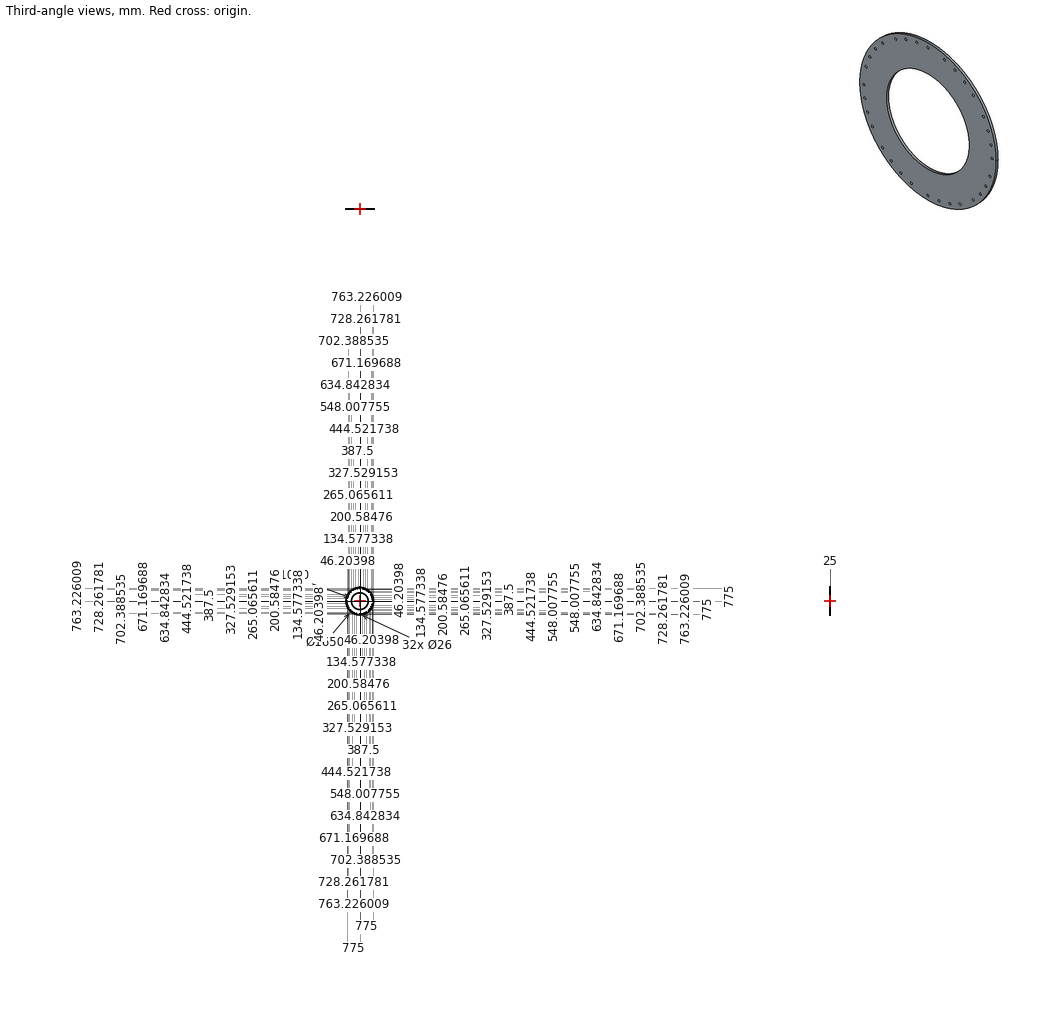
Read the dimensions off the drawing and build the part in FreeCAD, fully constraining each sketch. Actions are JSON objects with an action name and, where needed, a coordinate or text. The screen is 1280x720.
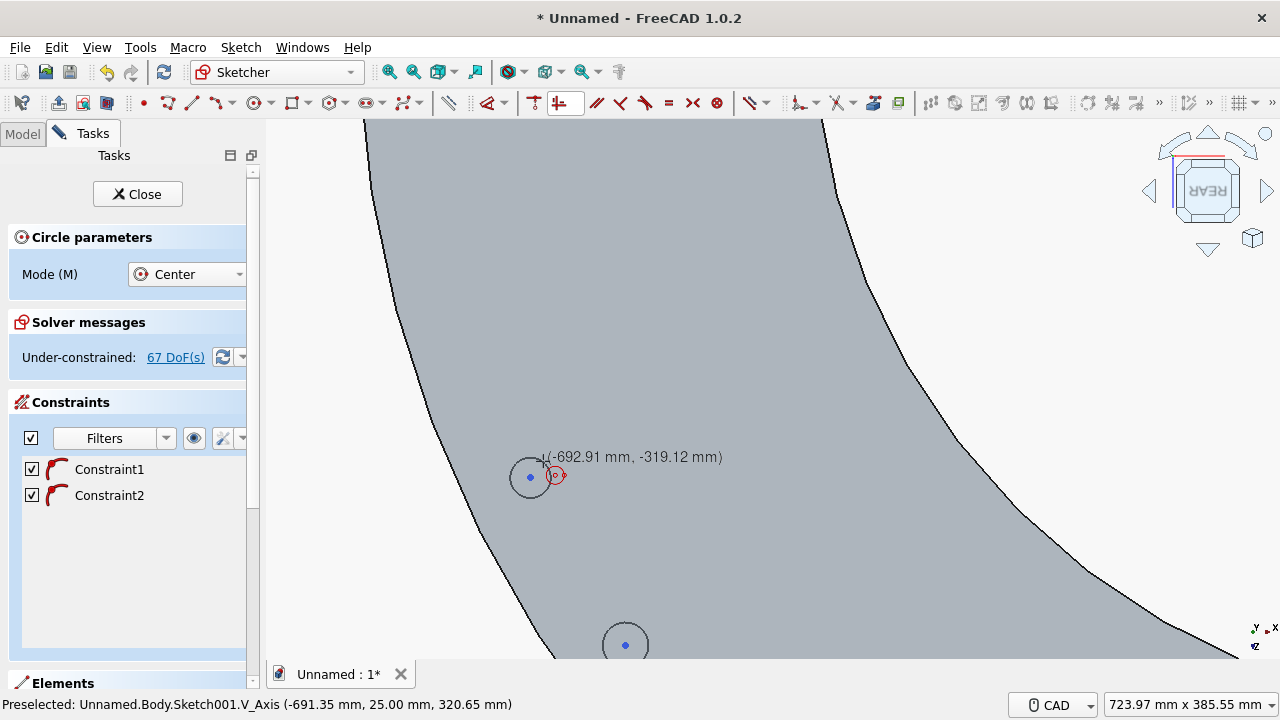
{"action": "scroll", "coordinate": [465, 296], "scroll_direction": "up", "scroll_amount": 2}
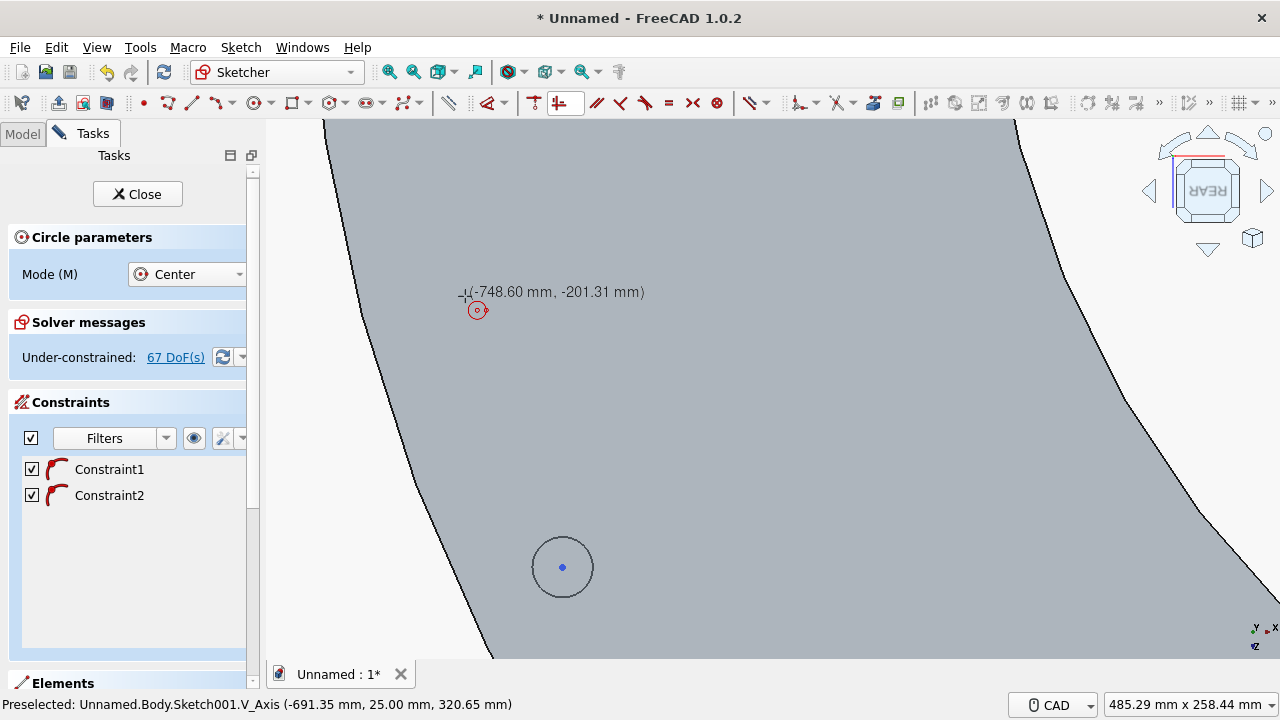
{"action": "scroll", "coordinate": [539, 453], "scroll_direction": "down", "scroll_amount": 11}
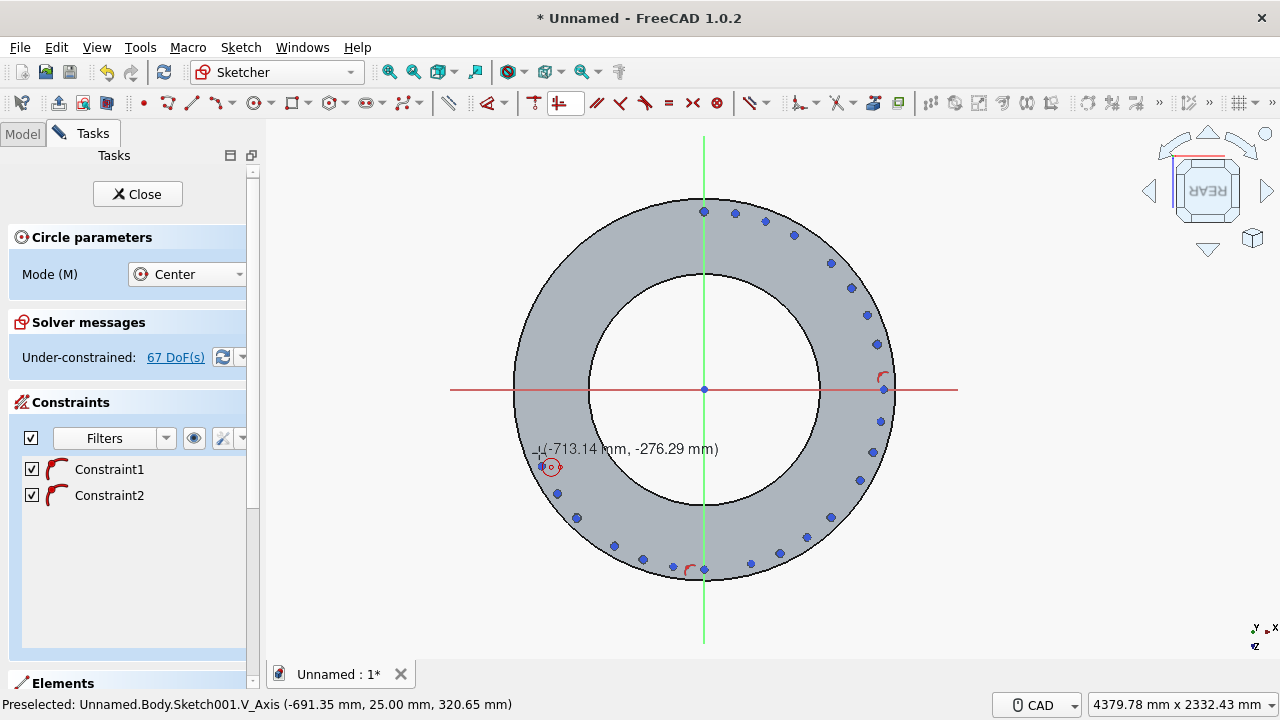
{"action": "left_click", "coordinate": [531, 436]}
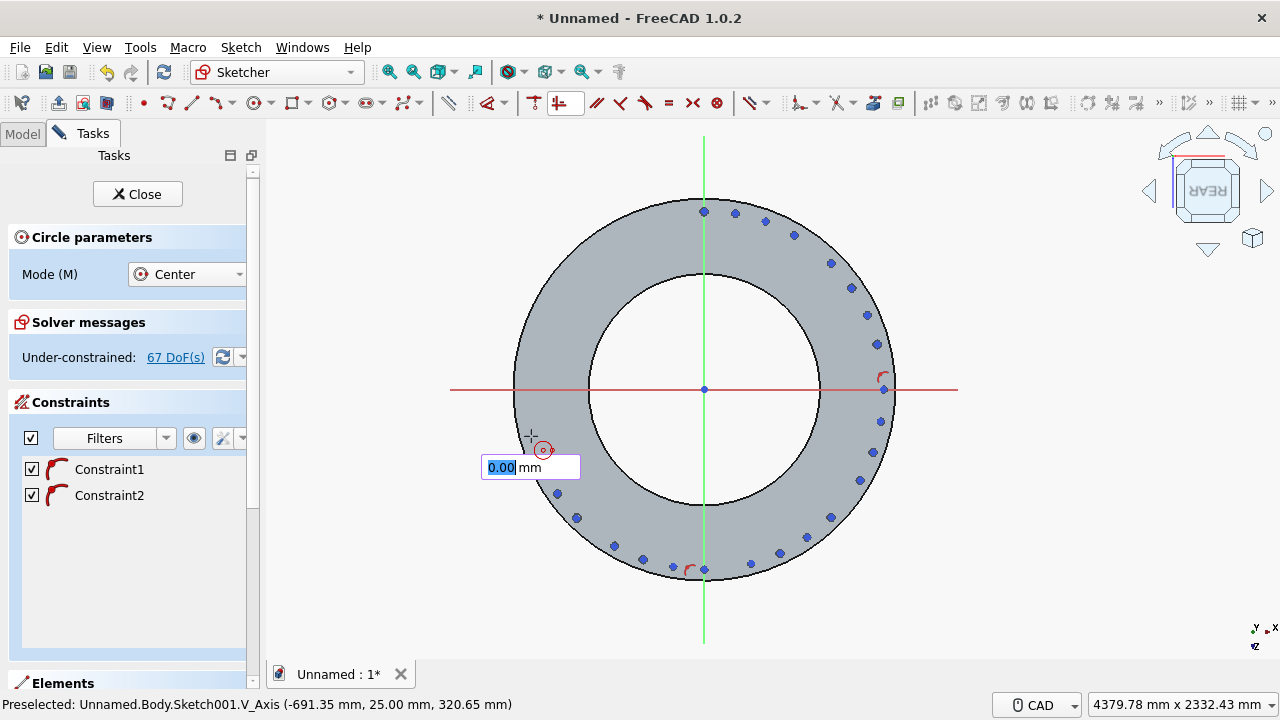
{"action": "scroll", "coordinate": [533, 434], "scroll_direction": "up", "scroll_amount": 9}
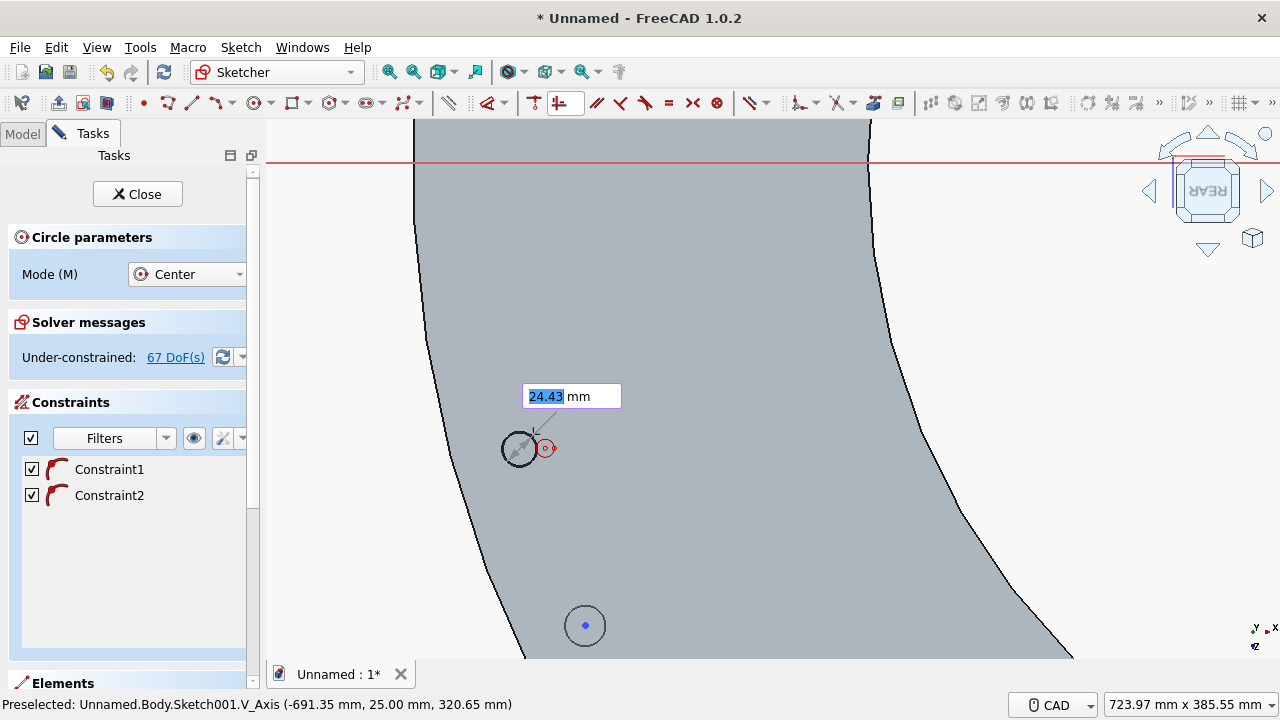
{"action": "left_click", "coordinate": [533, 431]}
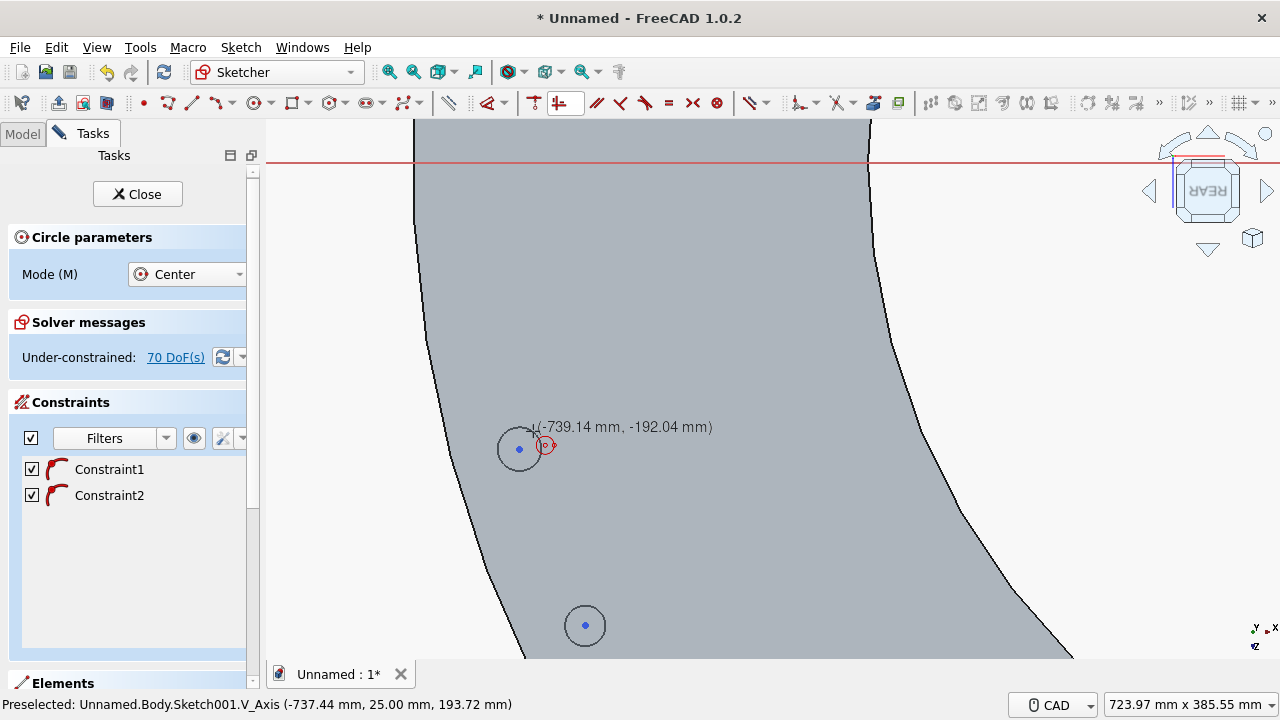
{"action": "scroll", "coordinate": [483, 163], "scroll_direction": "up", "scroll_amount": 2}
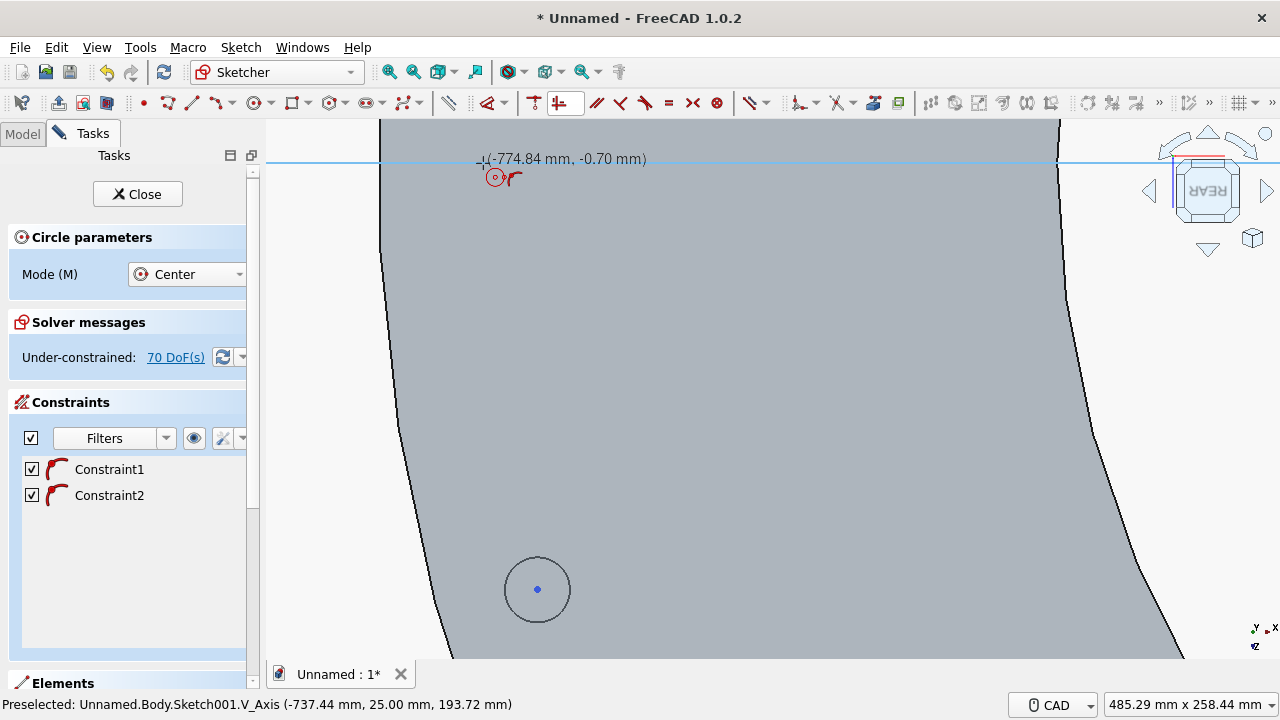
{"action": "scroll", "coordinate": [530, 417], "scroll_direction": "down", "scroll_amount": 11}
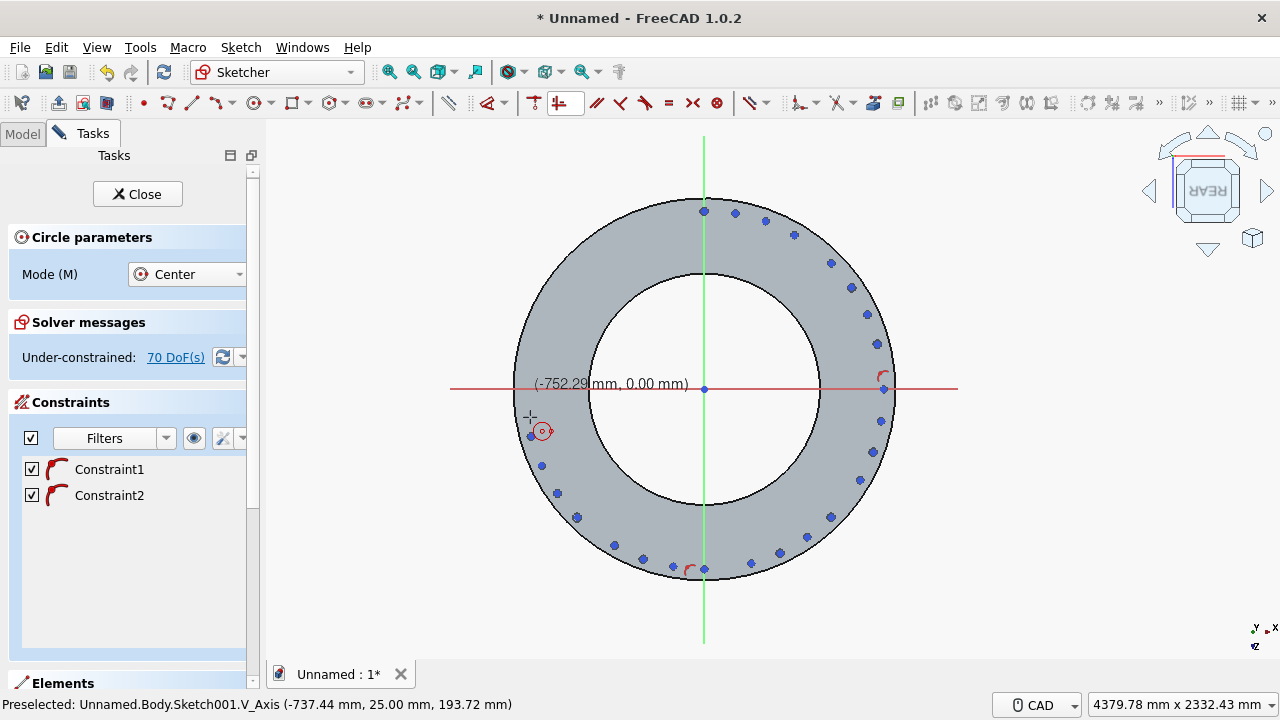
{"action": "left_click", "coordinate": [525, 389]}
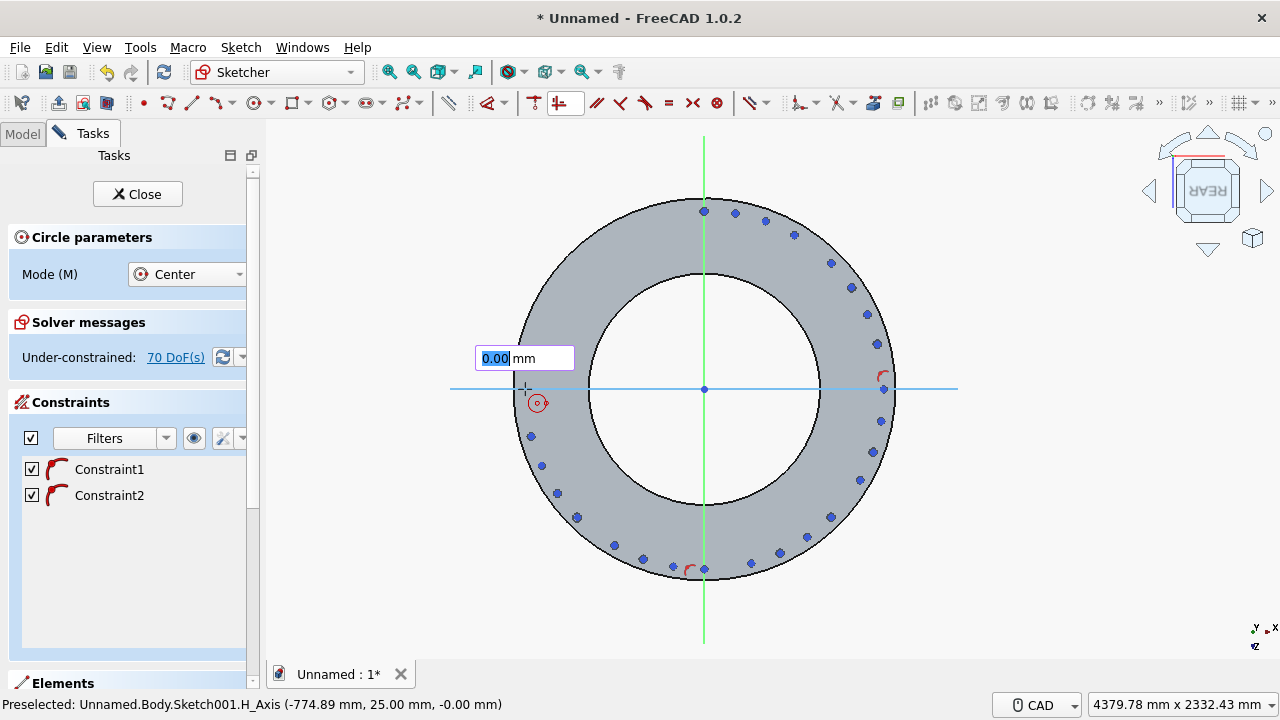
{"action": "scroll", "coordinate": [524, 392], "scroll_direction": "up", "scroll_amount": 9}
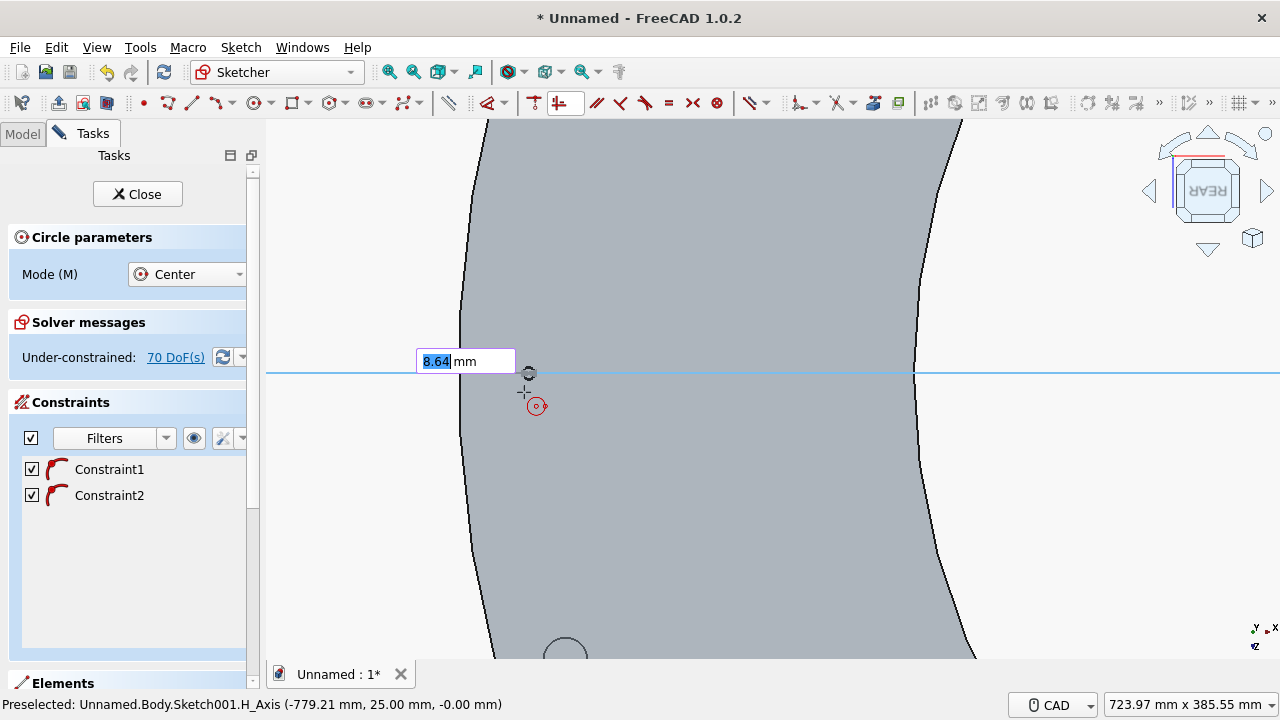
{"action": "left_click", "coordinate": [522, 391]}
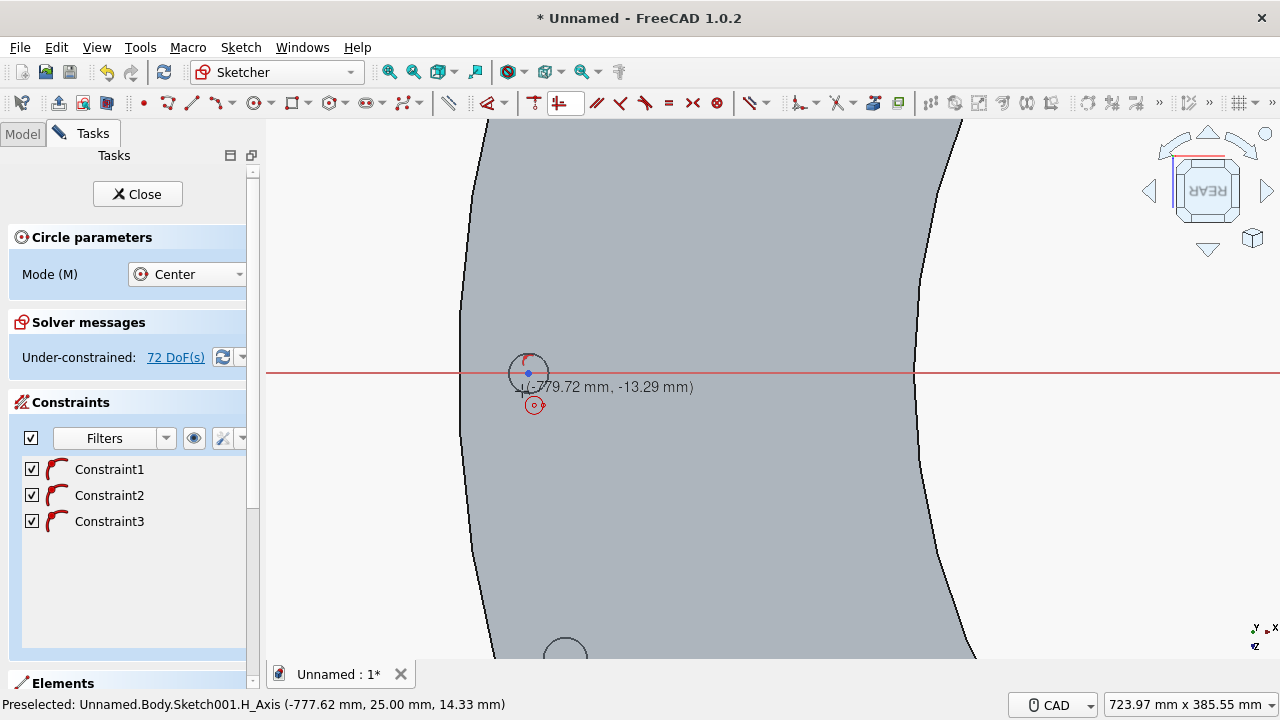
{"action": "scroll", "coordinate": [545, 185], "scroll_direction": "up", "scroll_amount": 2}